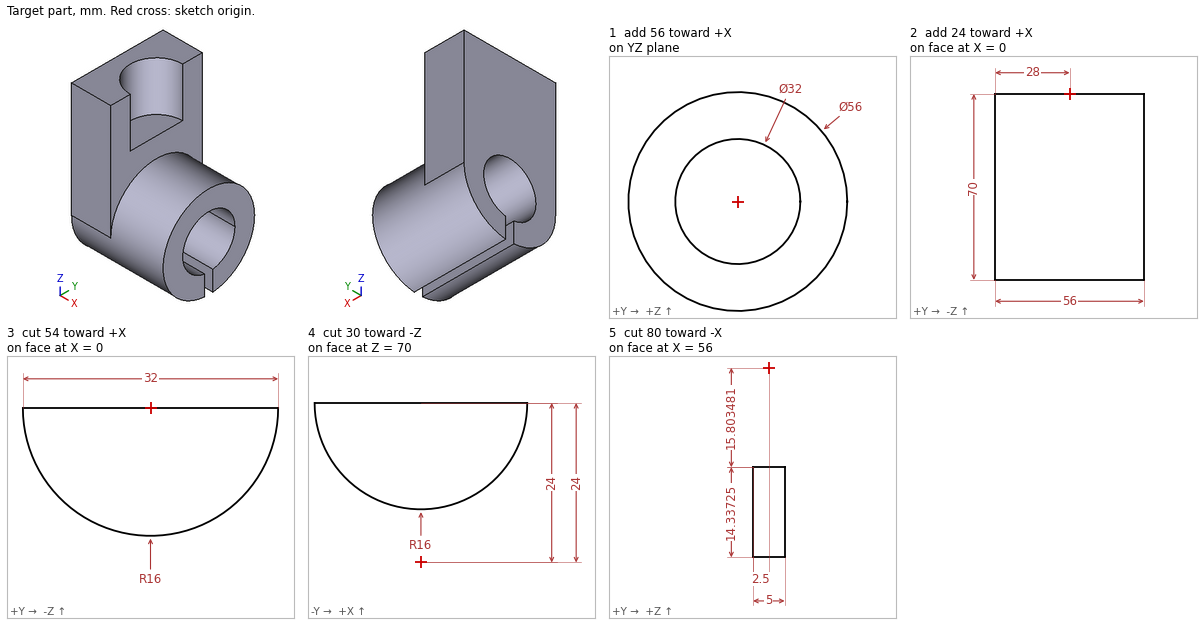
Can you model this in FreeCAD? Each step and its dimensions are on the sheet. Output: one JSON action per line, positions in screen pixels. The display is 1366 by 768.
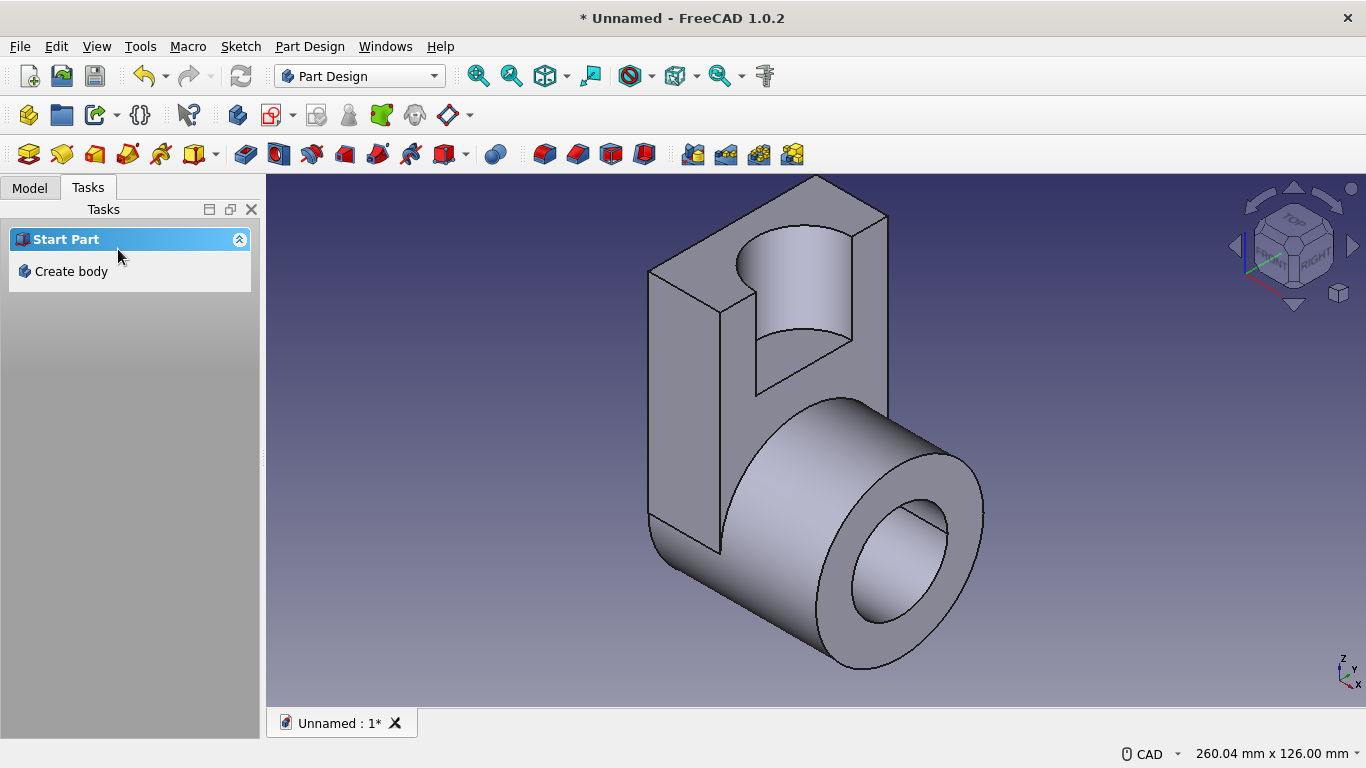
{"action": "left_click", "coordinate": [948, 588]}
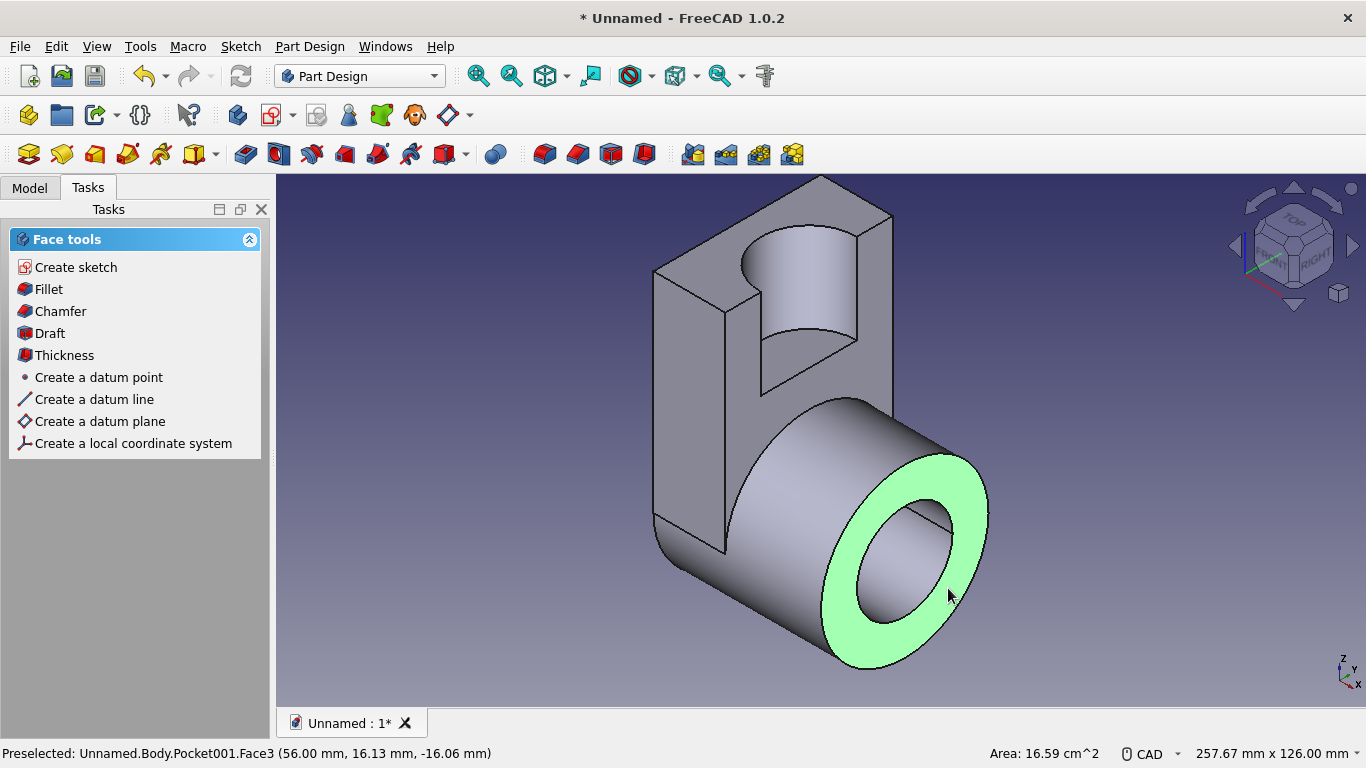
{"action": "left_click", "coordinate": [270, 116]}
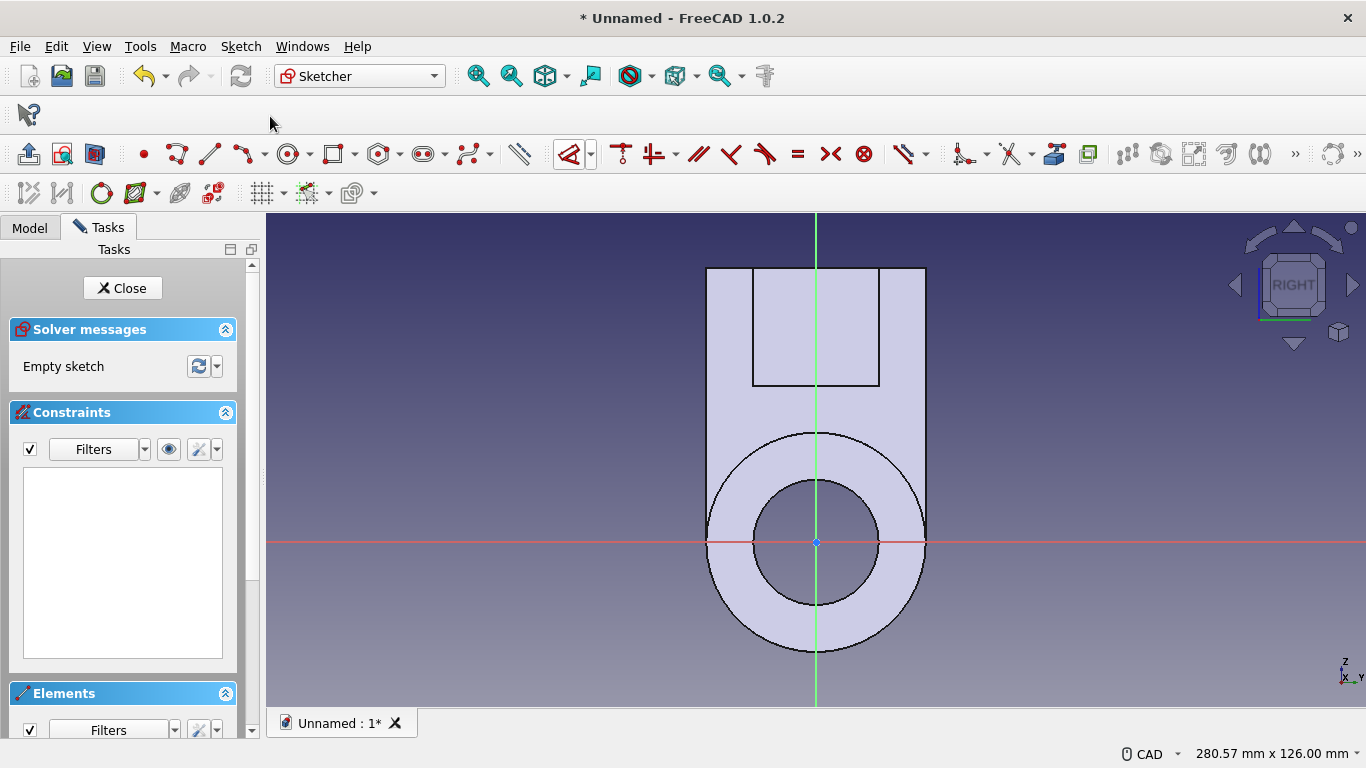
{"action": "scroll", "coordinate": [856, 679], "scroll_direction": "up", "scroll_amount": 5}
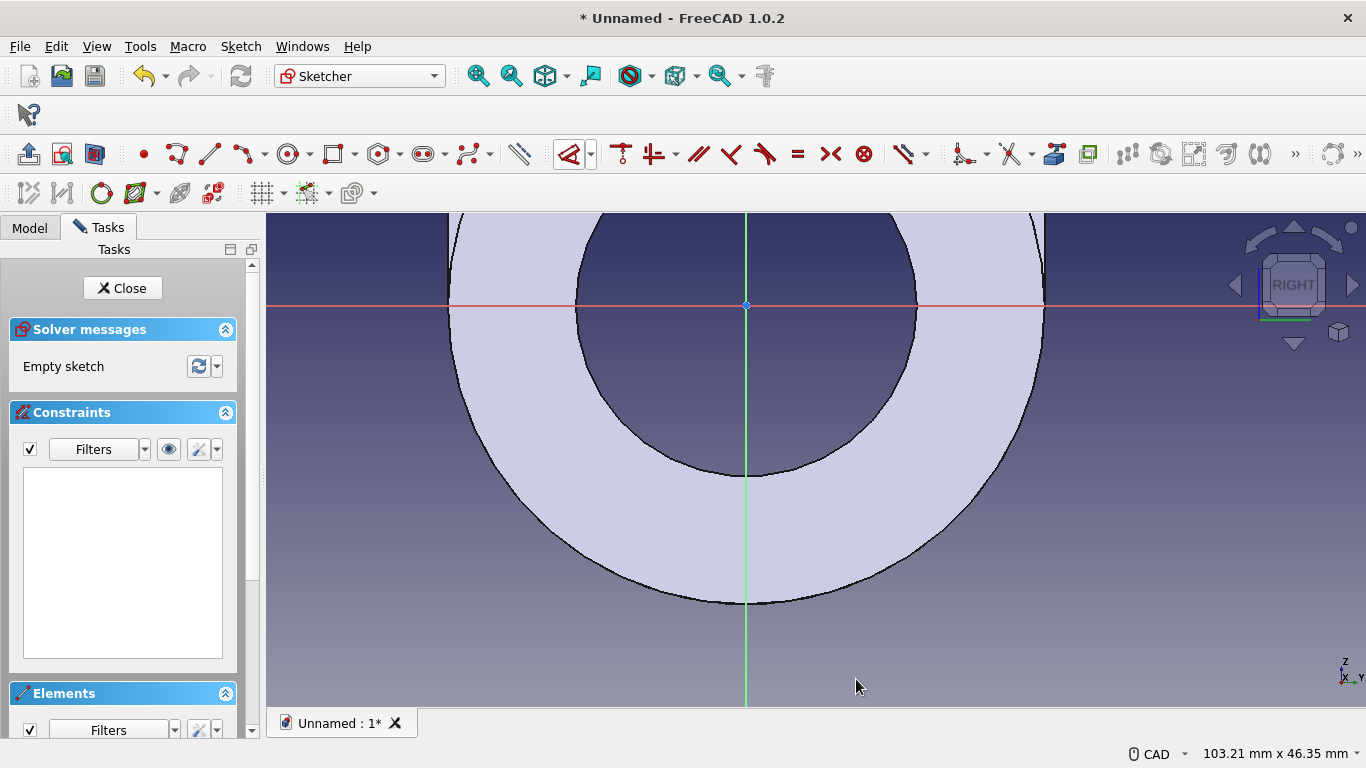
{"action": "left_click", "coordinate": [332, 154]}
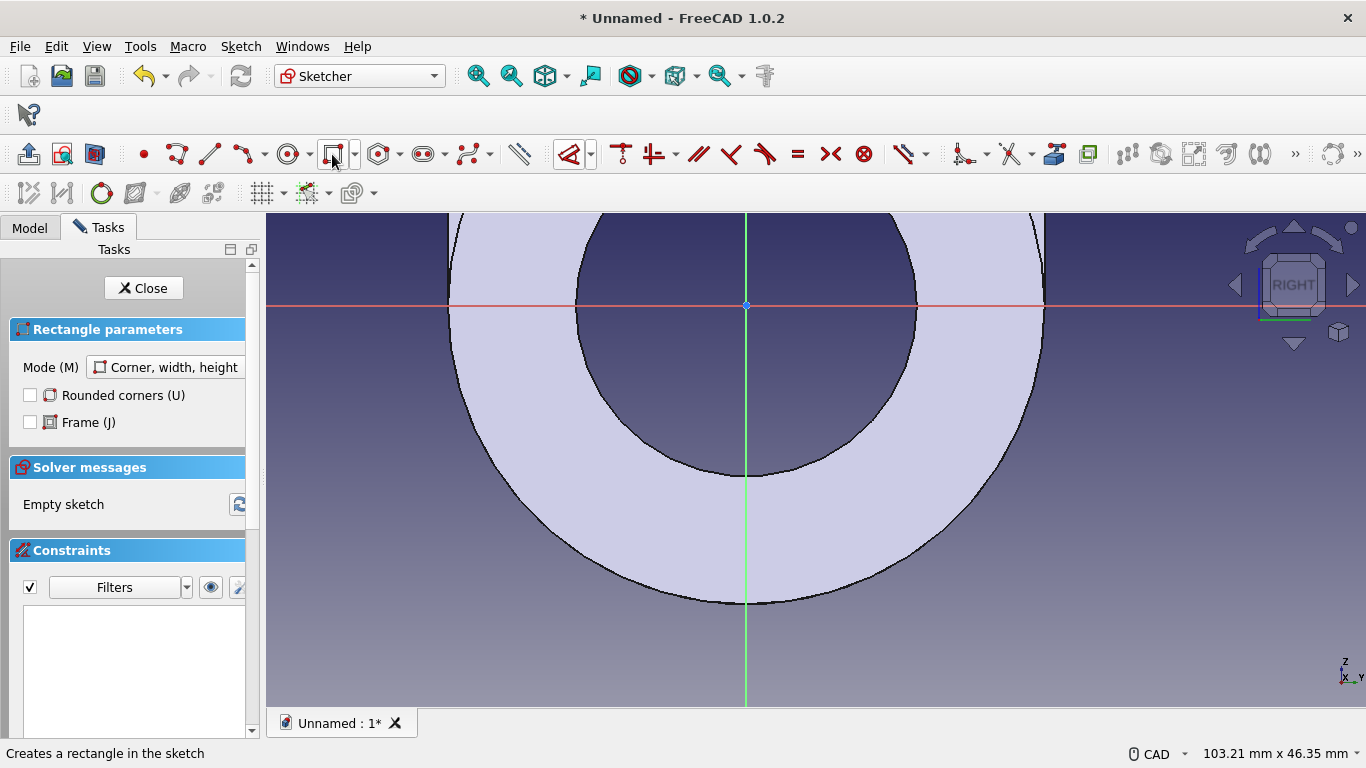
{"action": "left_click", "coordinate": [720, 474]}
{"action": "left_click", "coordinate": [773, 627]}
{"action": "key", "text": "Escape"}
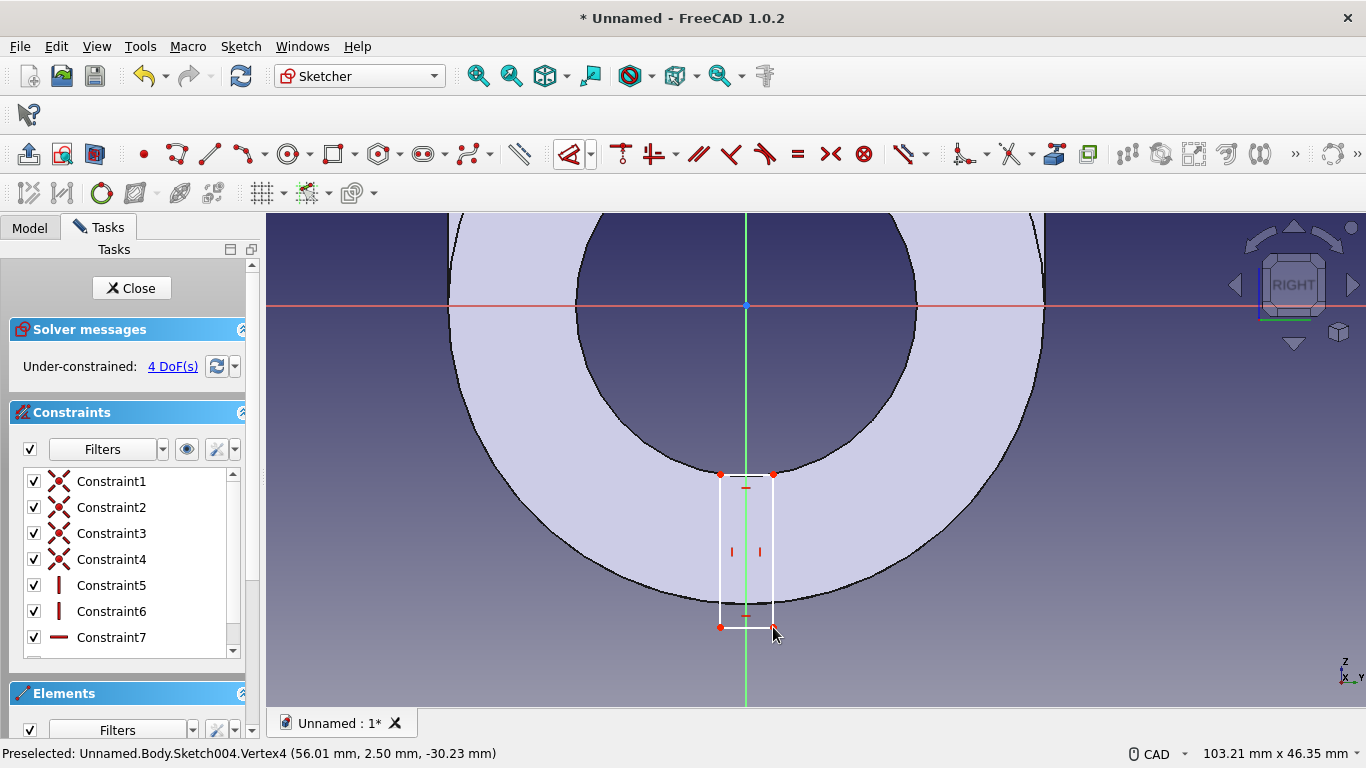
{"action": "scroll", "coordinate": [736, 628], "scroll_direction": "up", "scroll_amount": 2}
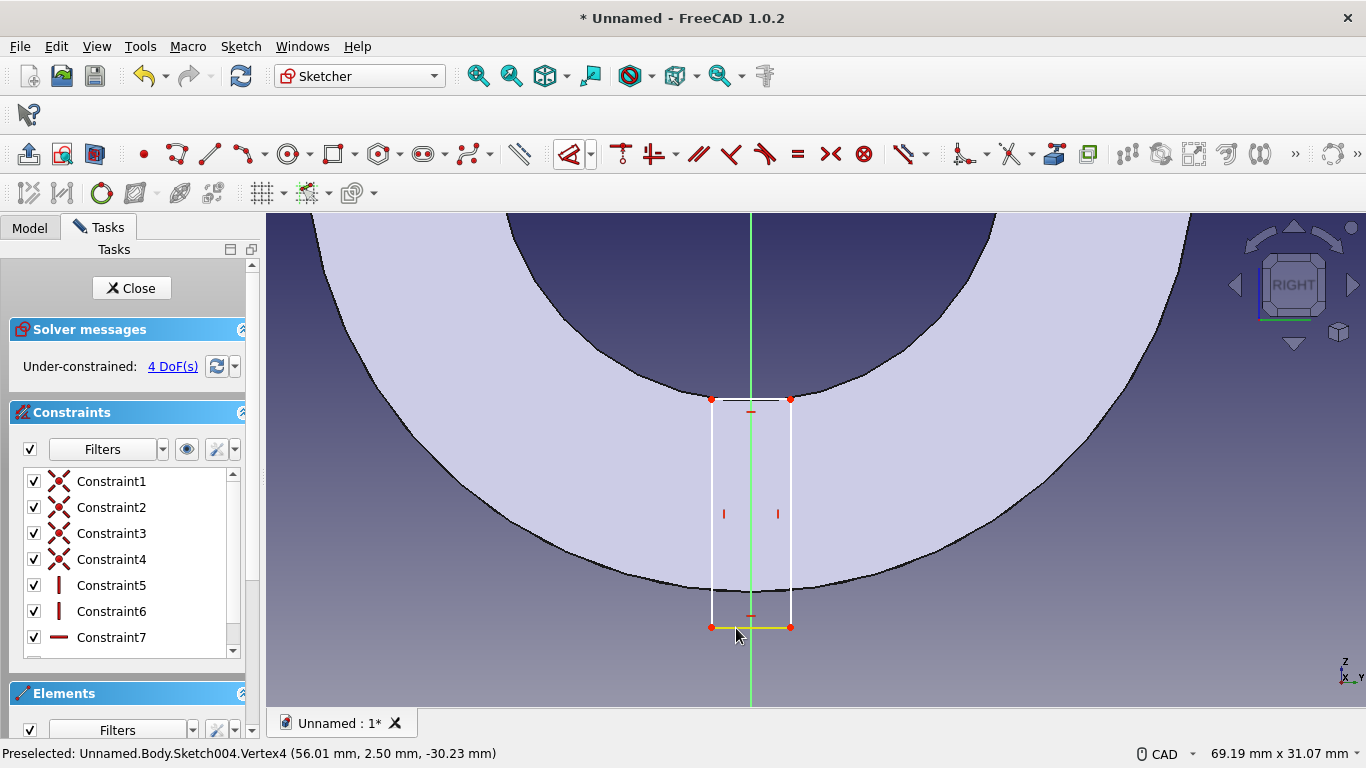
{"action": "left_click", "coordinate": [736, 628]}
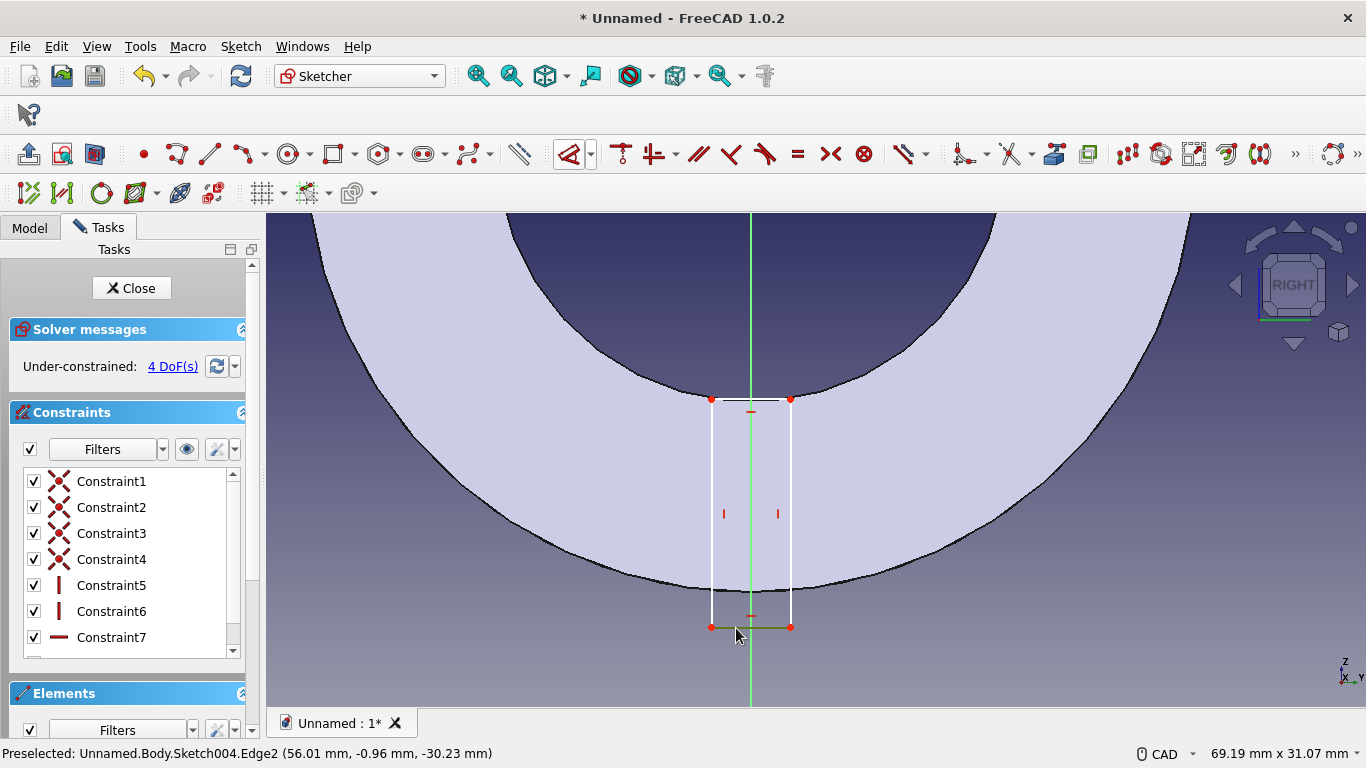
{"action": "left_click", "coordinate": [590, 154]}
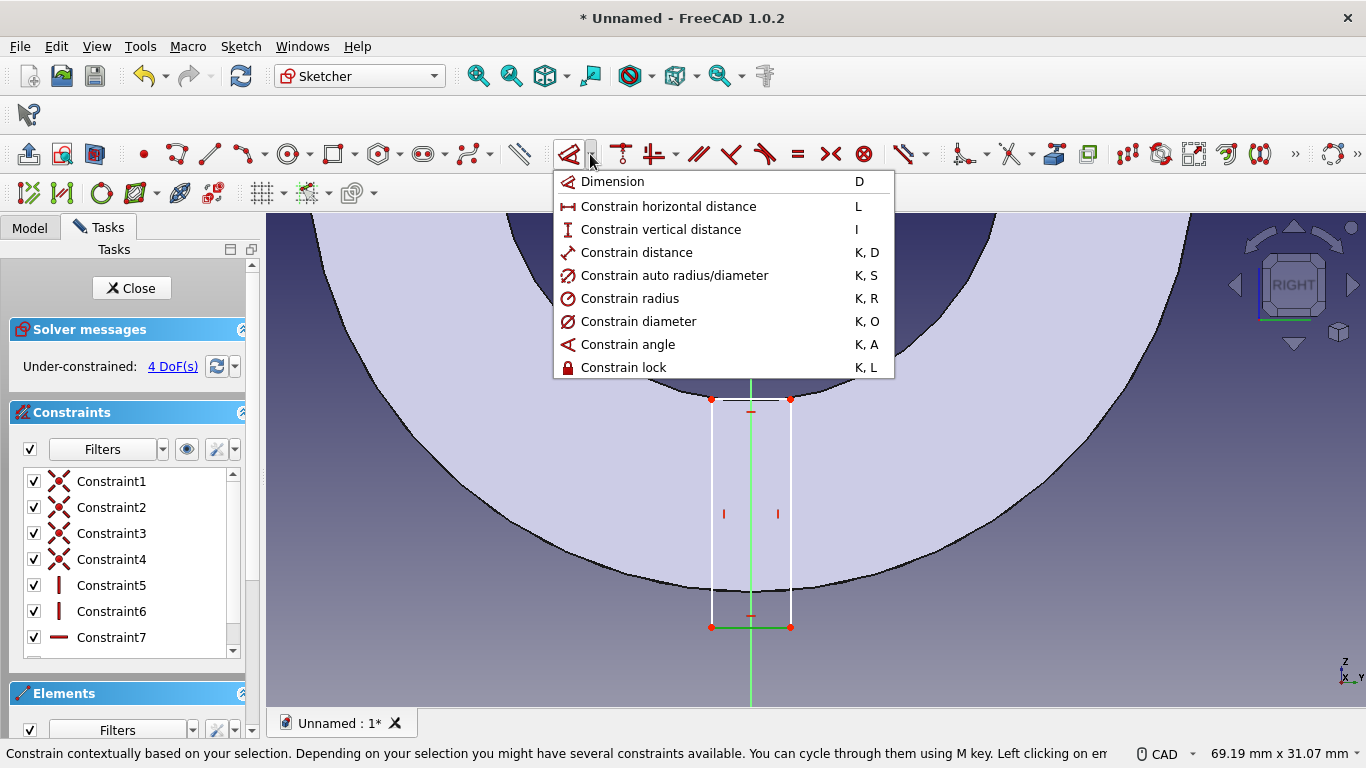
{"action": "left_click", "coordinate": [724, 206]}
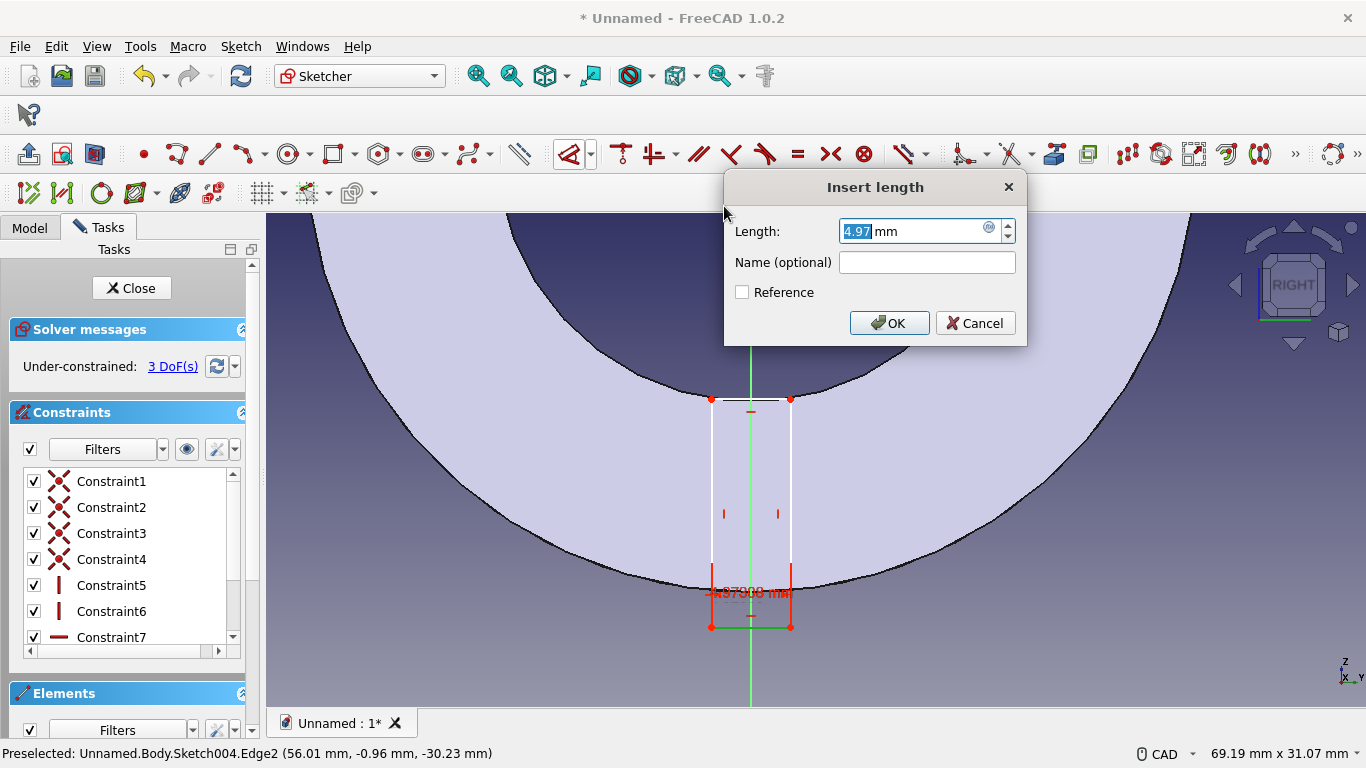
{"action": "type", "text": "5"}
{"action": "key", "text": "Return"}